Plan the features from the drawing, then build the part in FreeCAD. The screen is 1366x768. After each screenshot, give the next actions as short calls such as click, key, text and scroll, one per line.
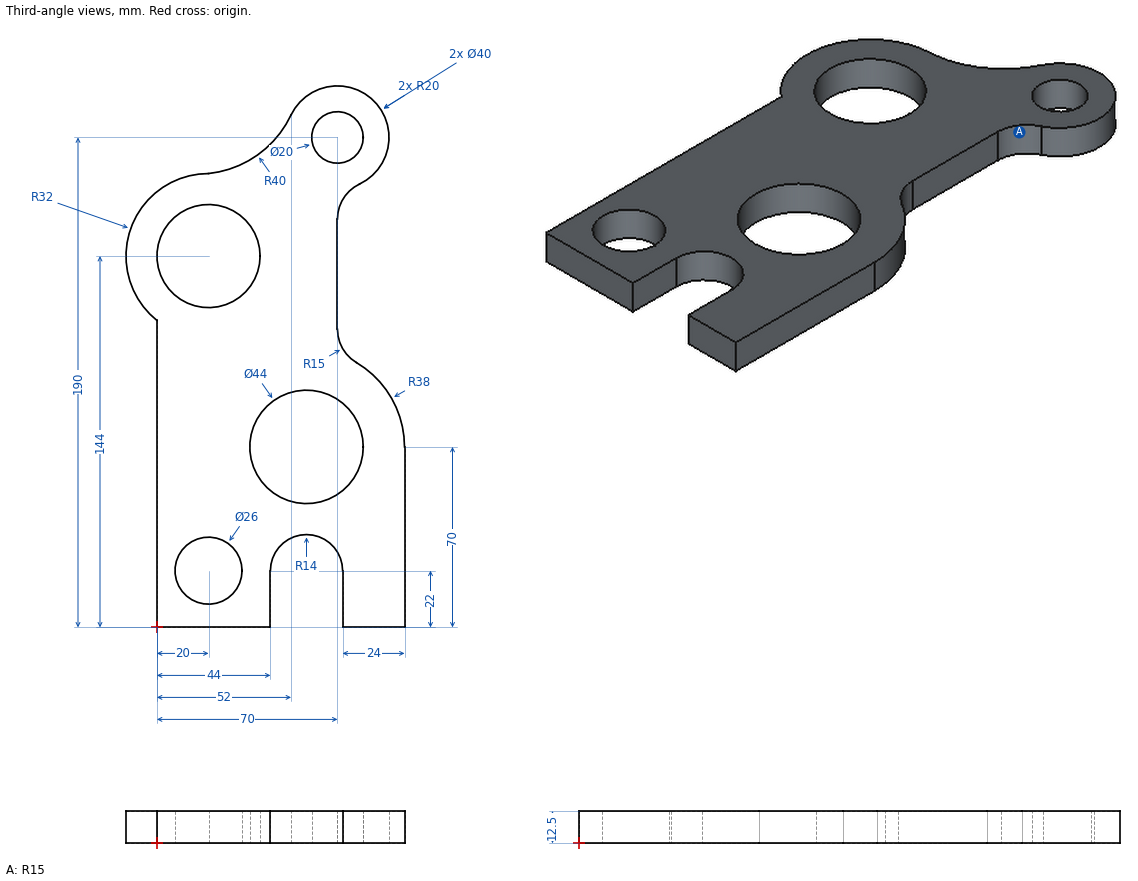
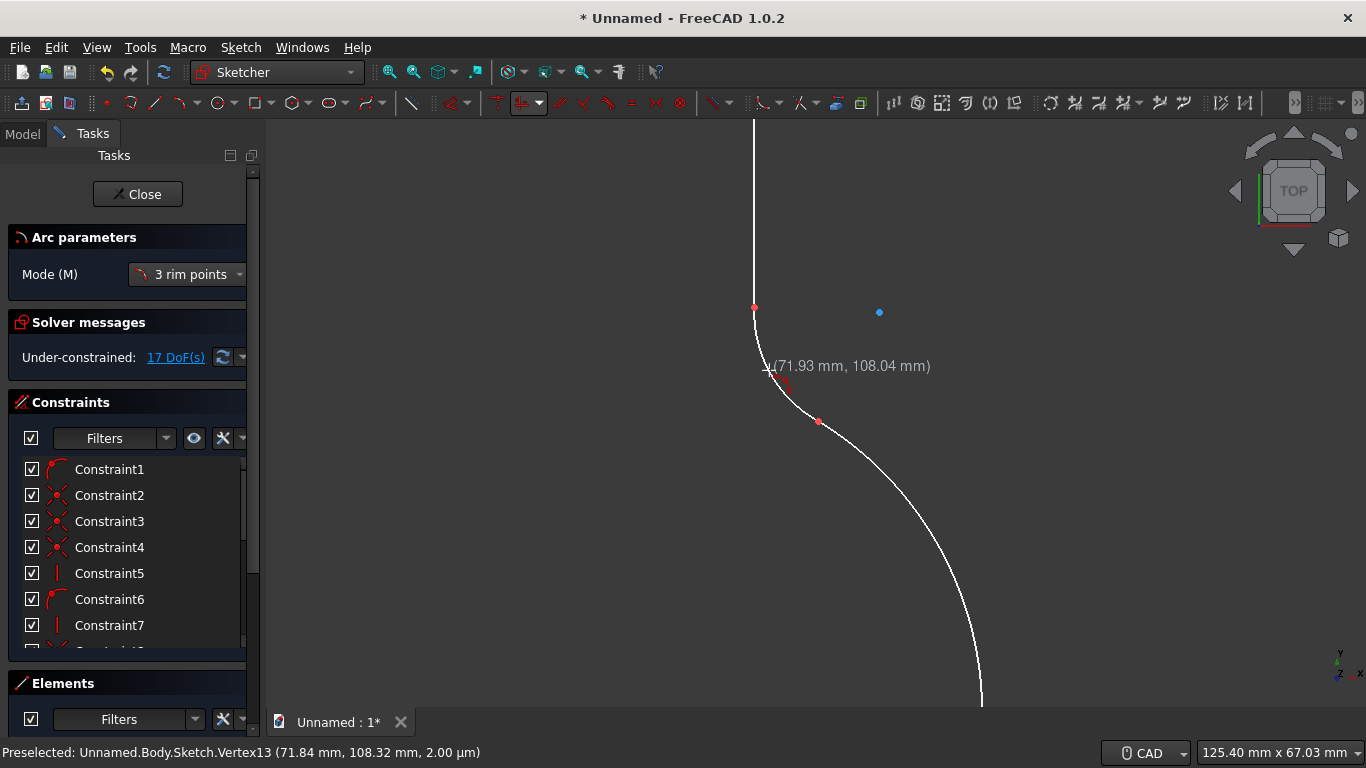
scroll(806, 406, down, 8)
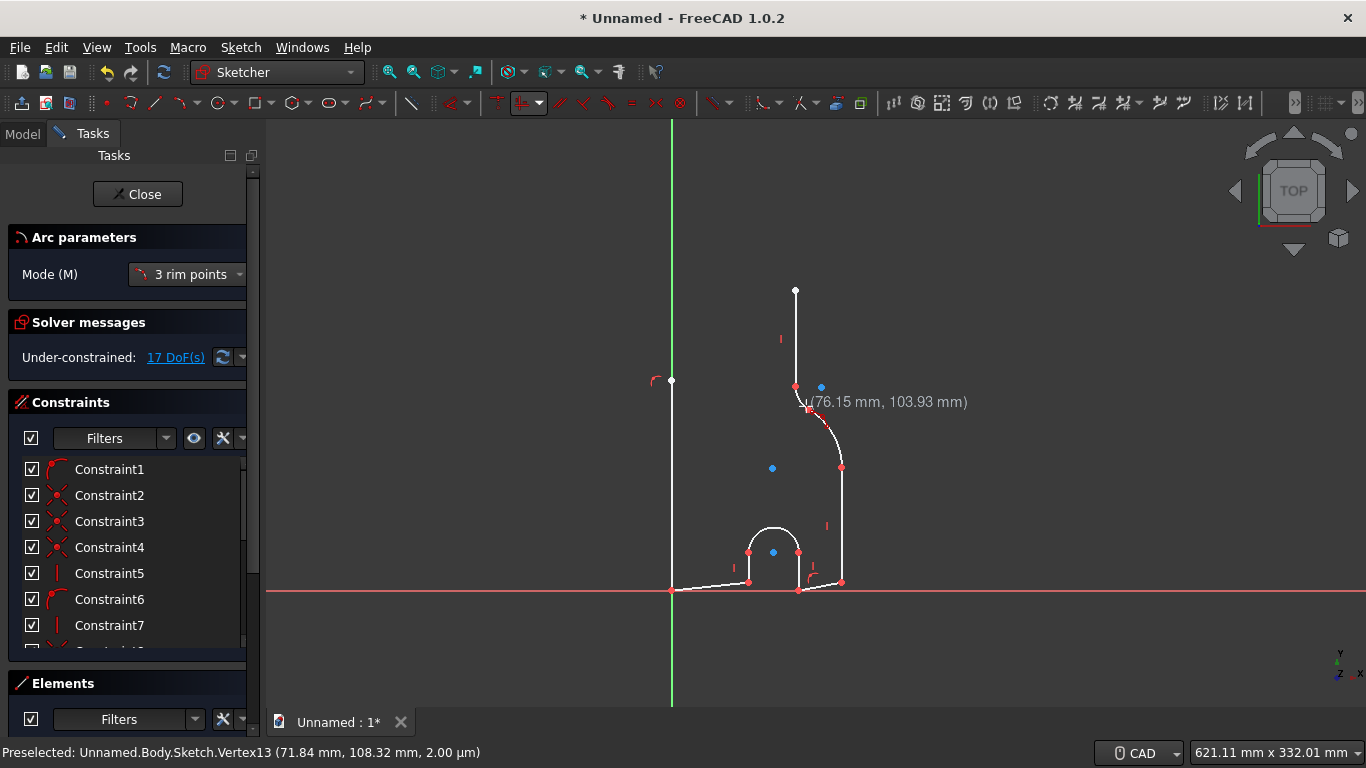
click(796, 291)
click(764, 239)
click(826, 235)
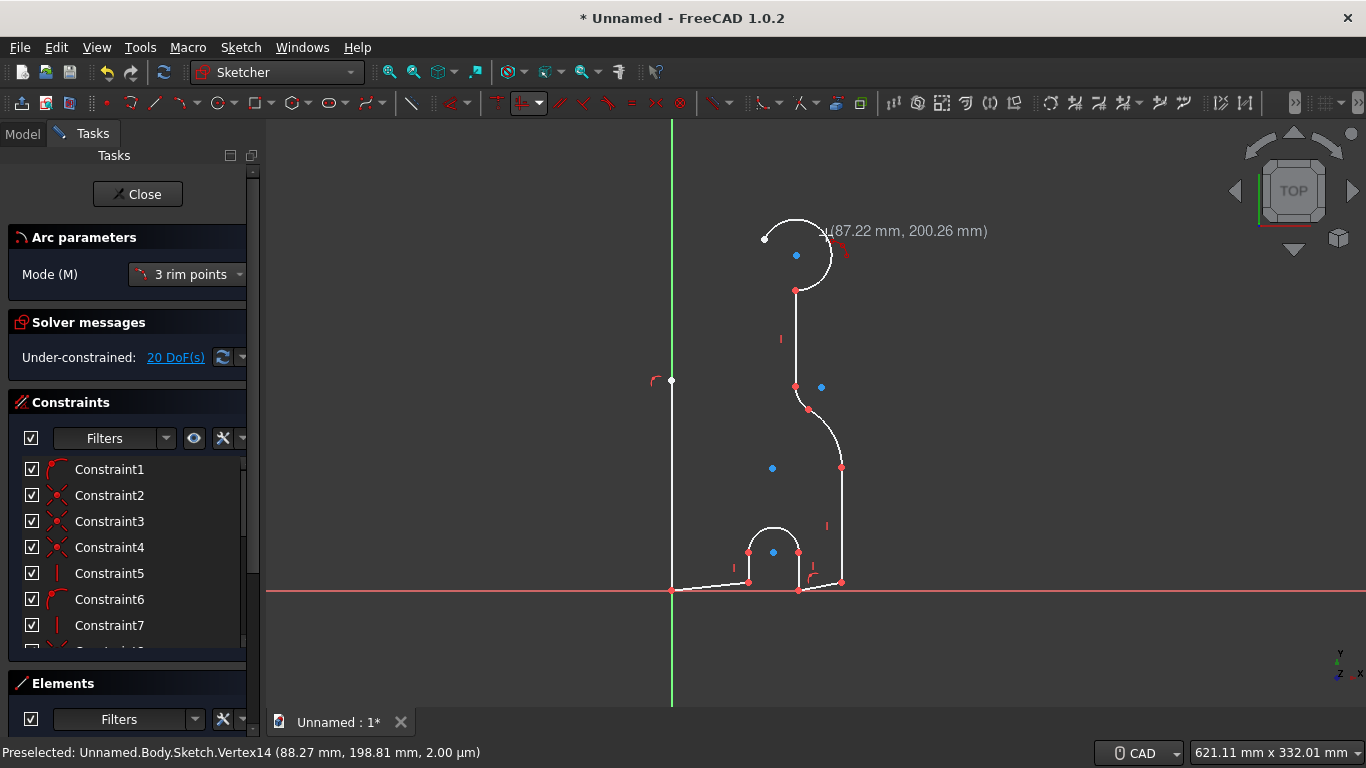
click(764, 240)
click(707, 279)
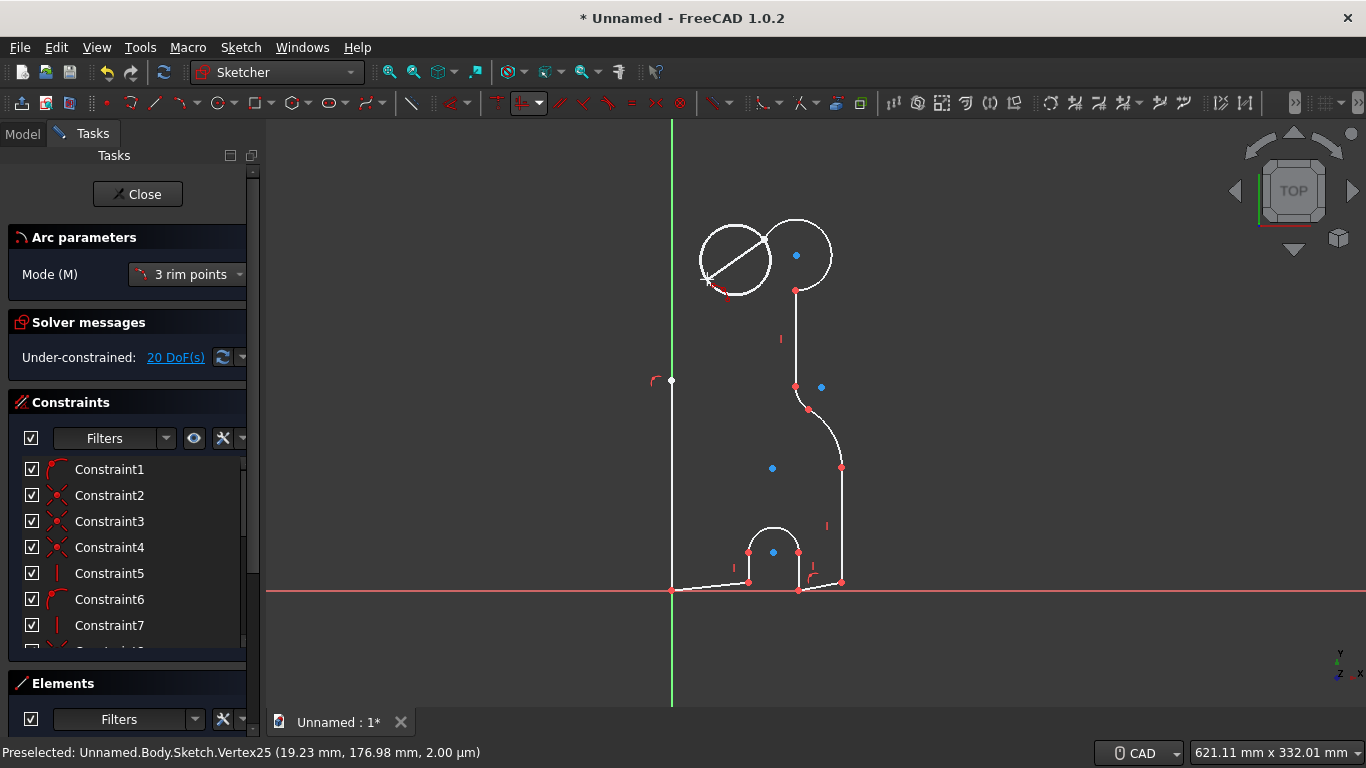
scroll(741, 266, up, 3)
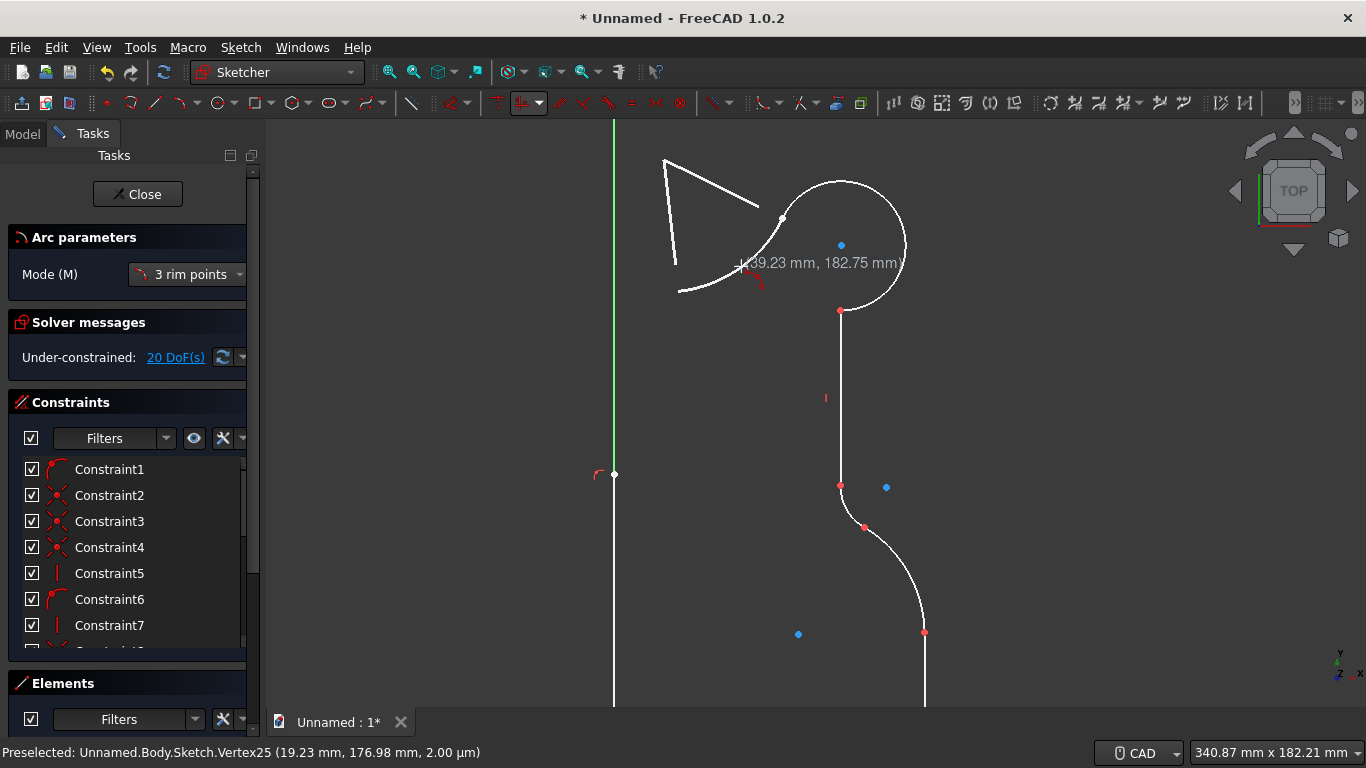
click(740, 266)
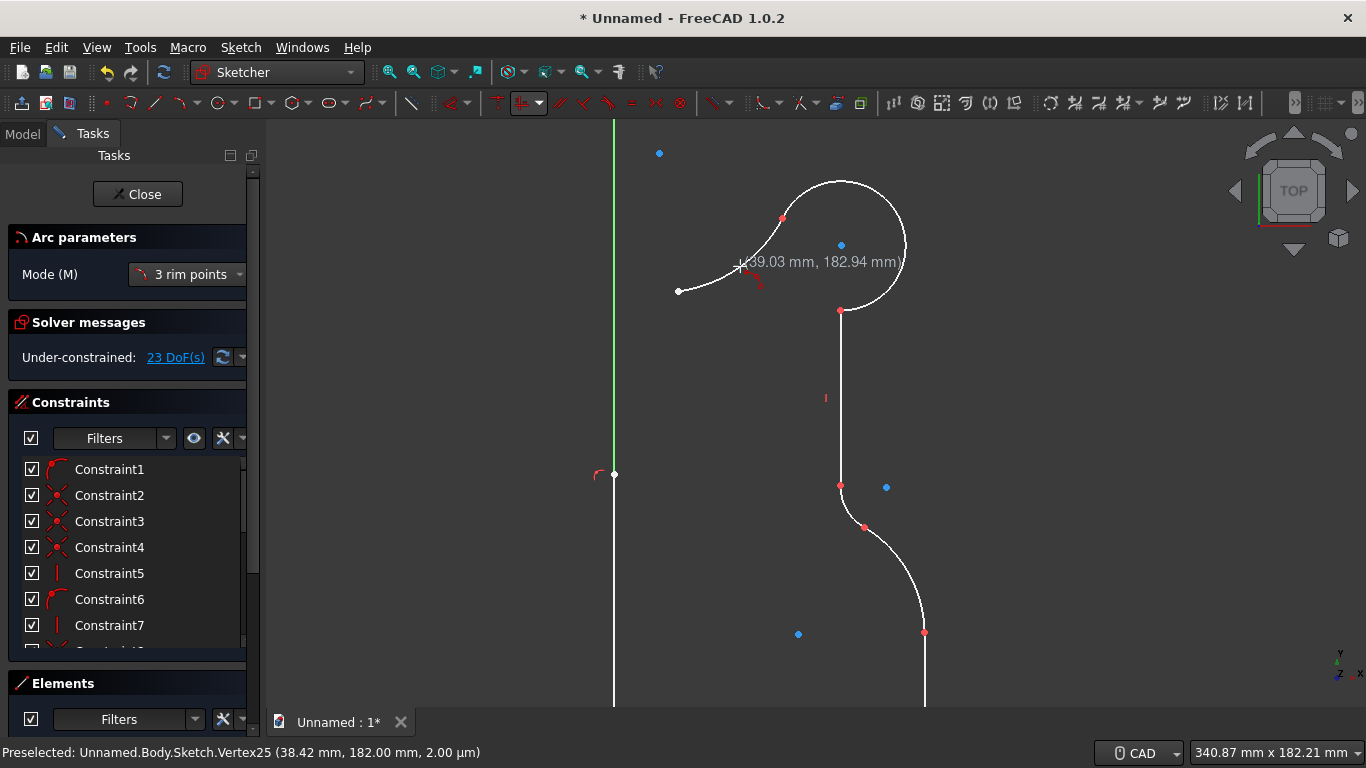
click(679, 291)
click(614, 474)
click(581, 358)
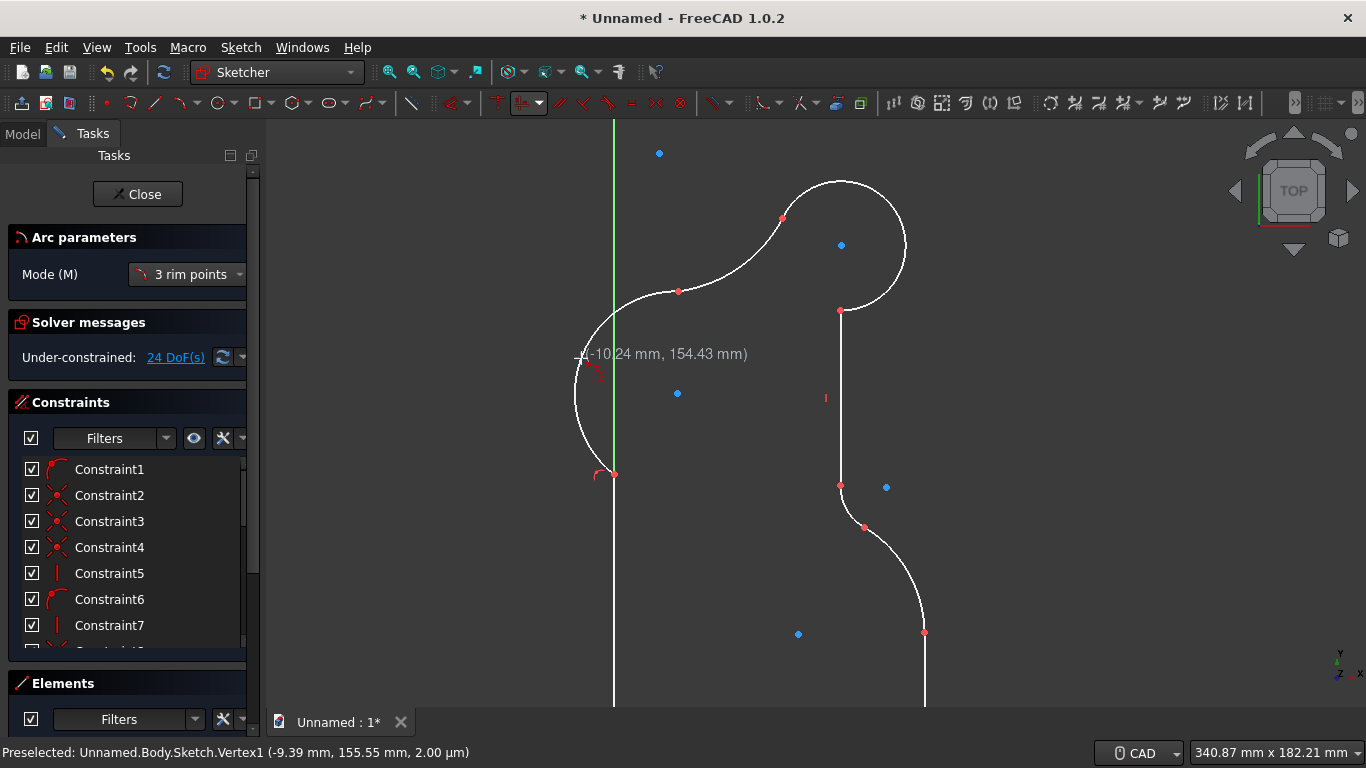
click(218, 104)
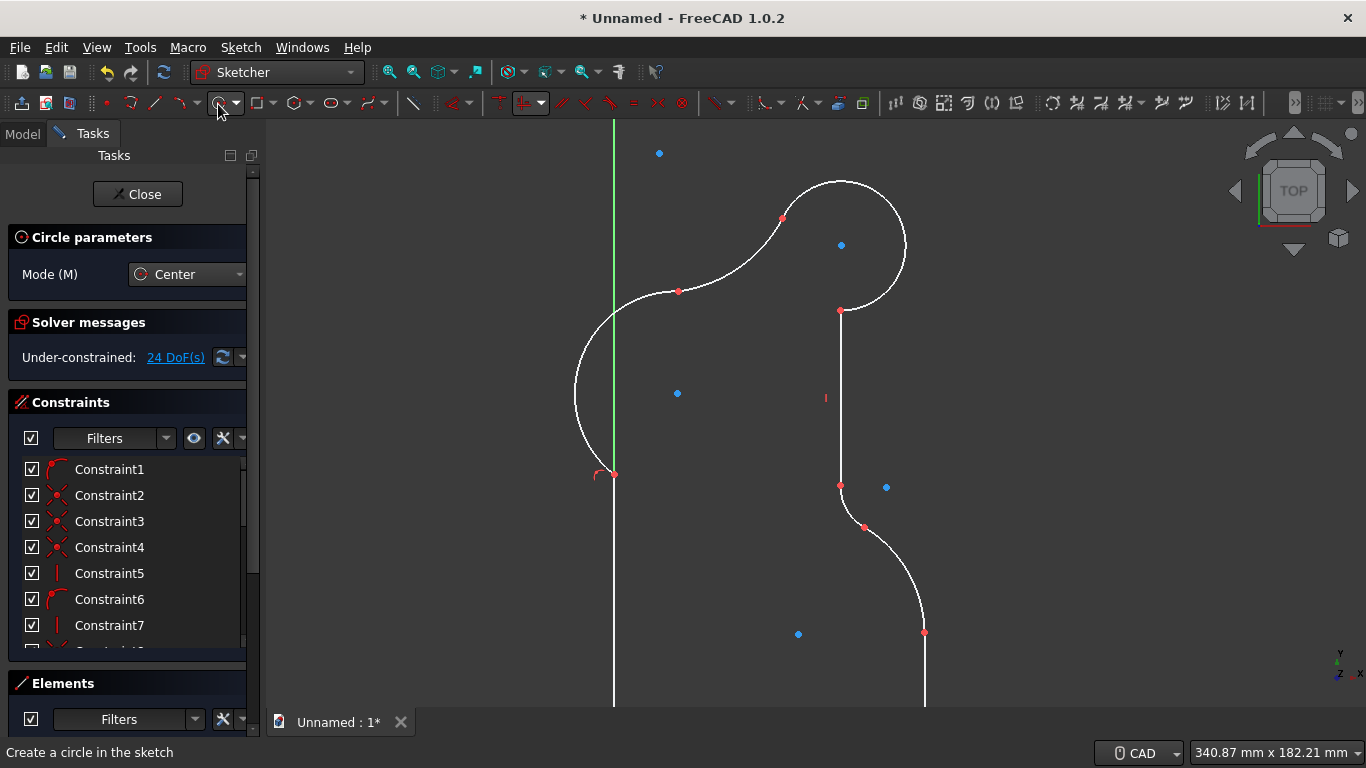
scroll(741, 266, down, 3)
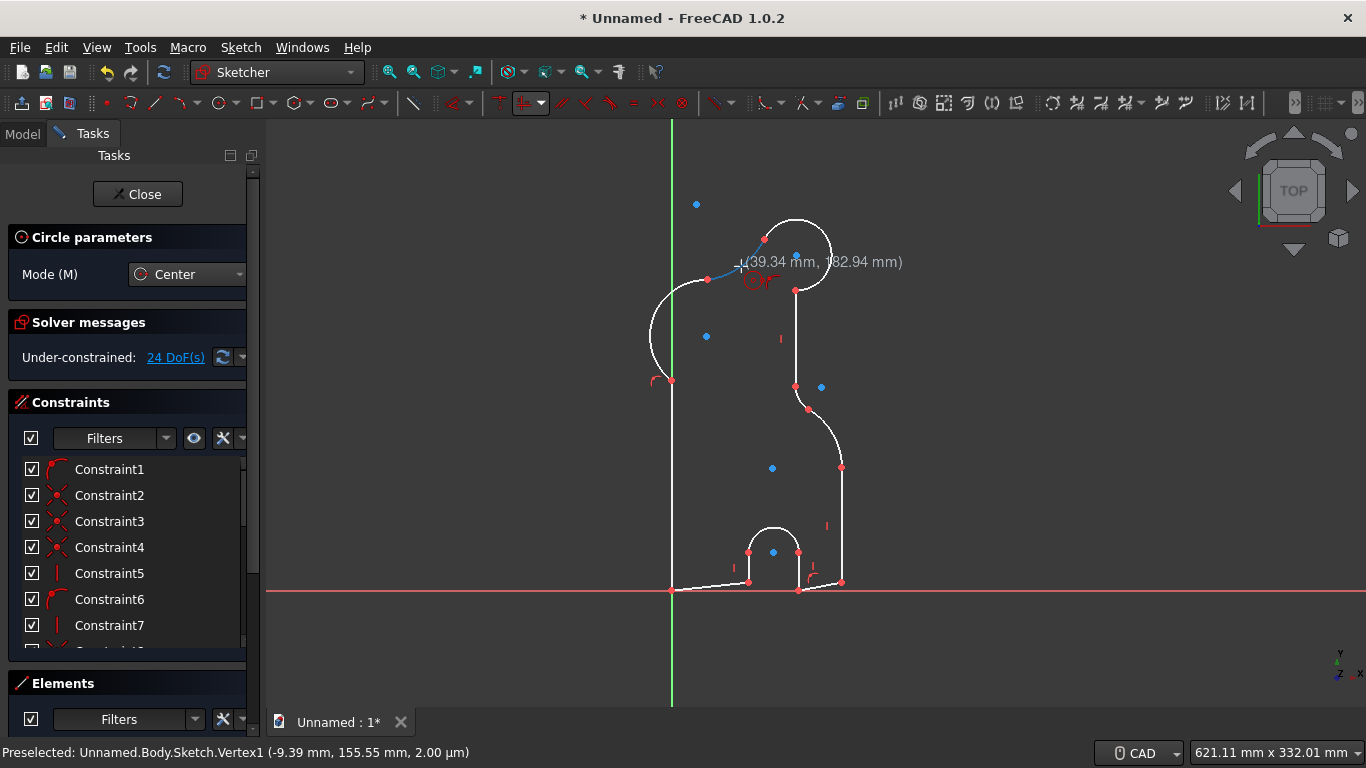
click(707, 552)
click(723, 535)